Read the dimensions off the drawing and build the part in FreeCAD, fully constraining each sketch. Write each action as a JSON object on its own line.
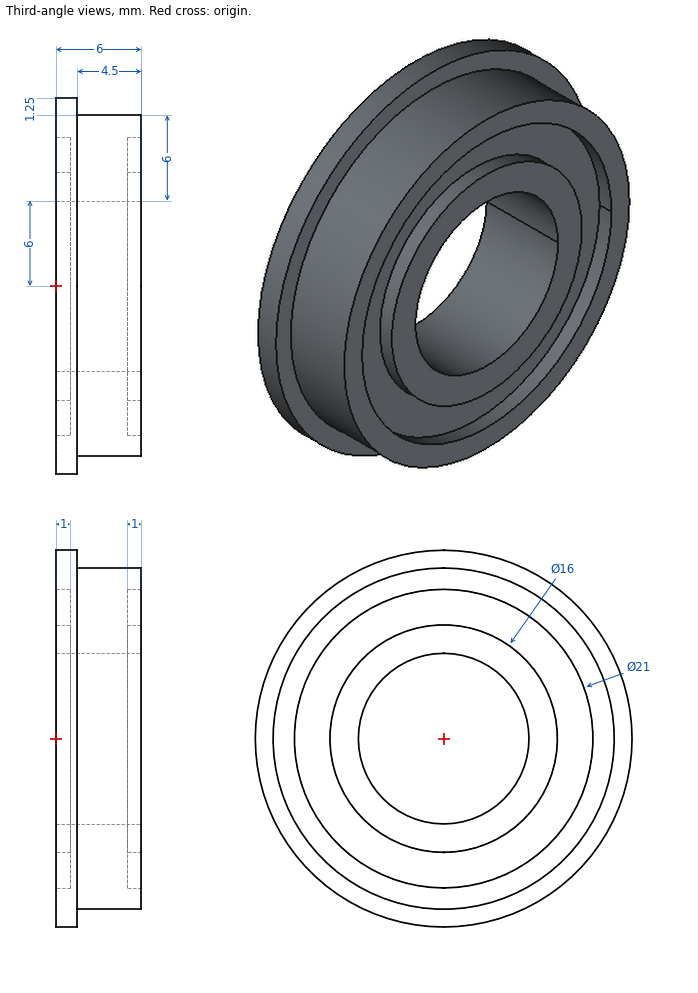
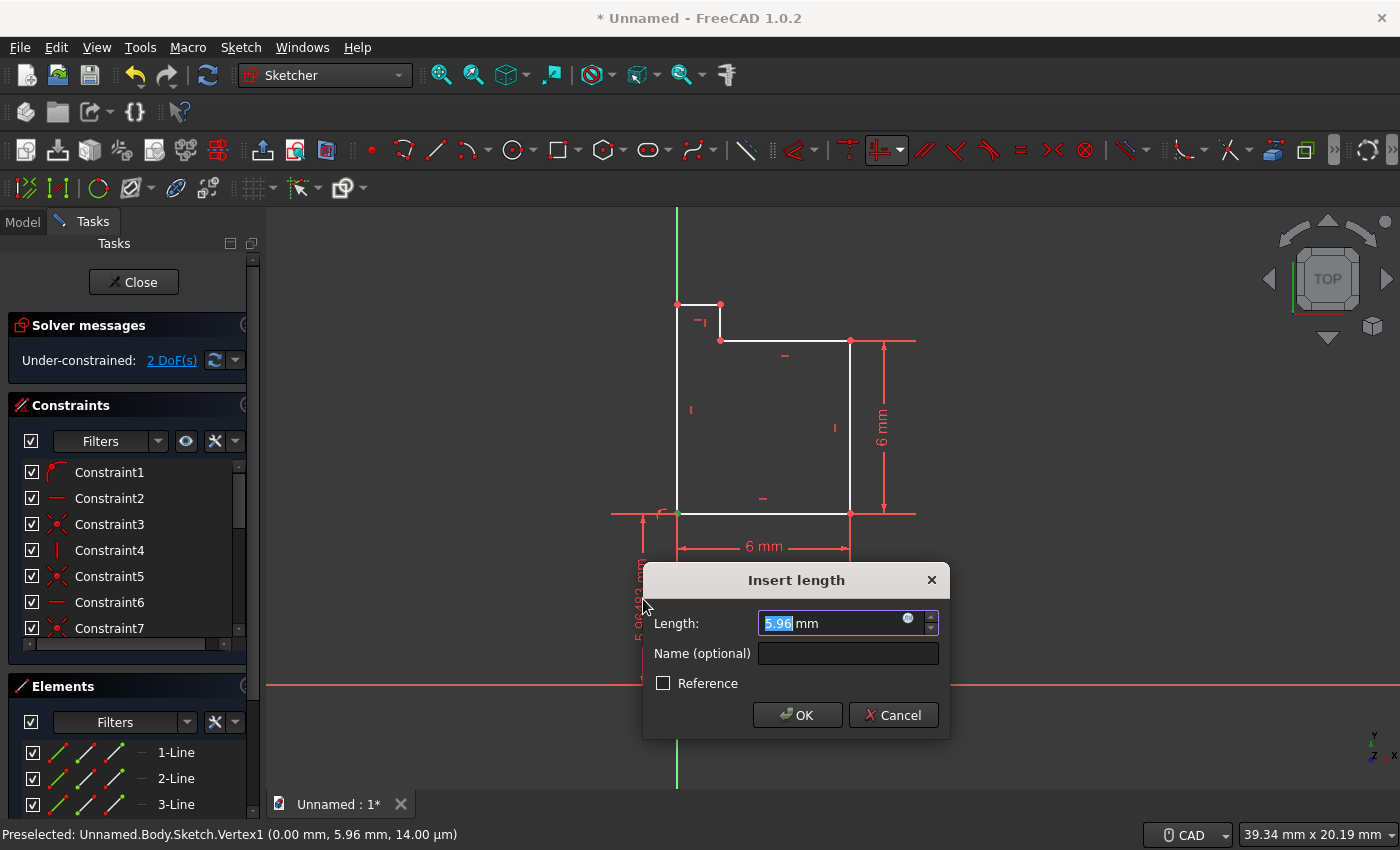
{"action": "type", "text": "6"}
{"action": "key", "text": "Return"}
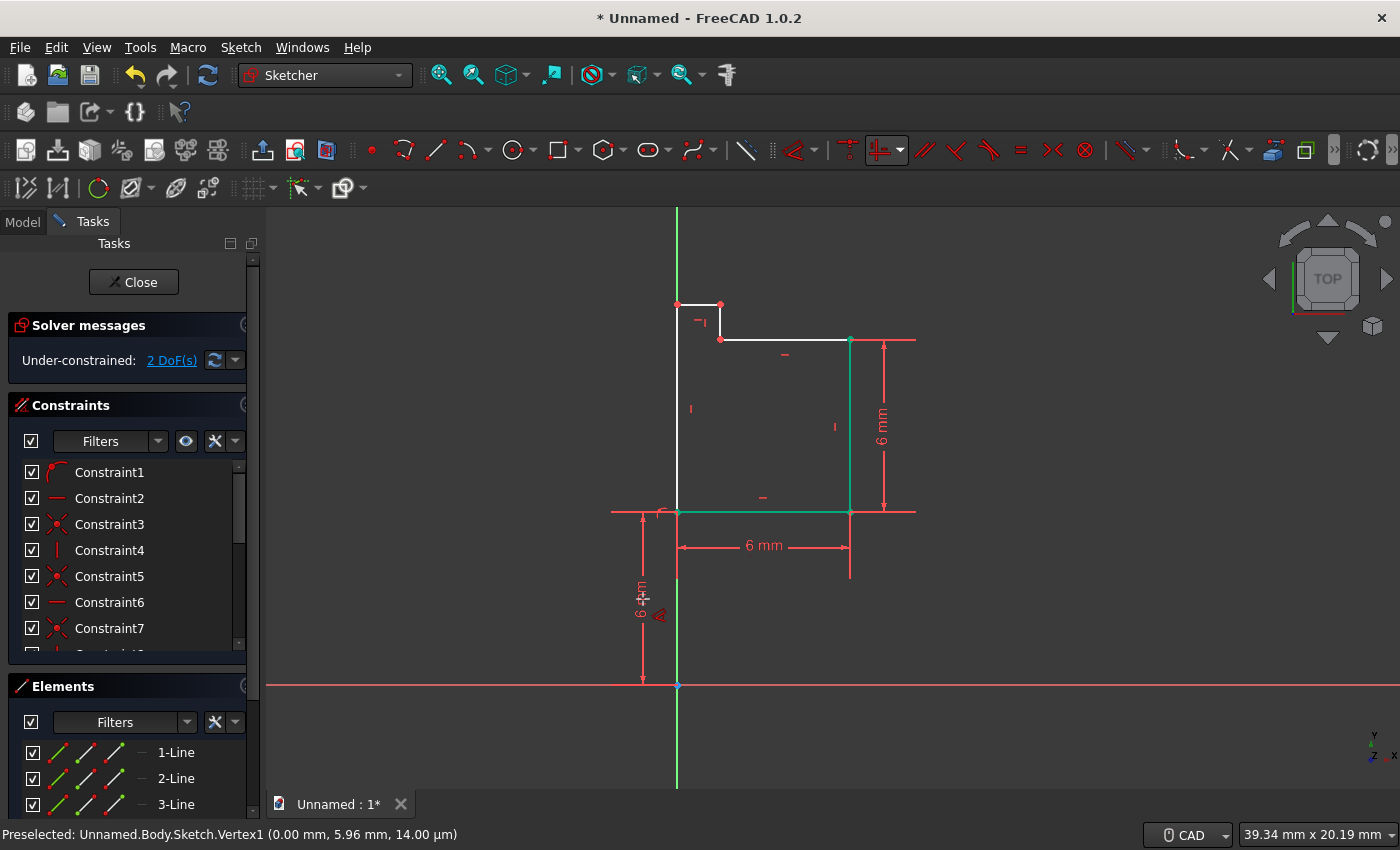
{"action": "left_click", "coordinate": [811, 340]}
{"action": "left_click", "coordinate": [785, 306]}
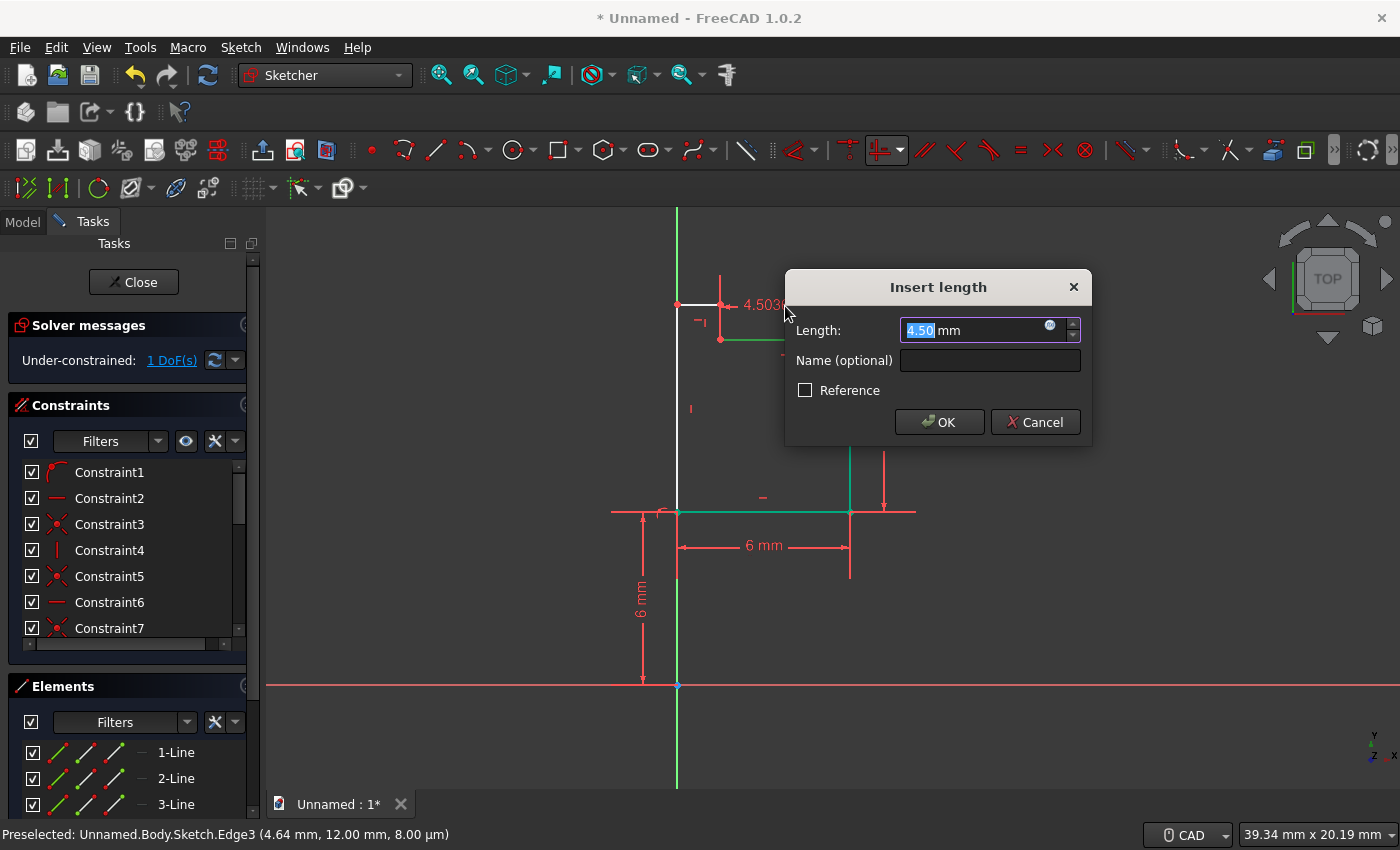
{"action": "type", "text": "4.5"}
{"action": "key", "text": "Return"}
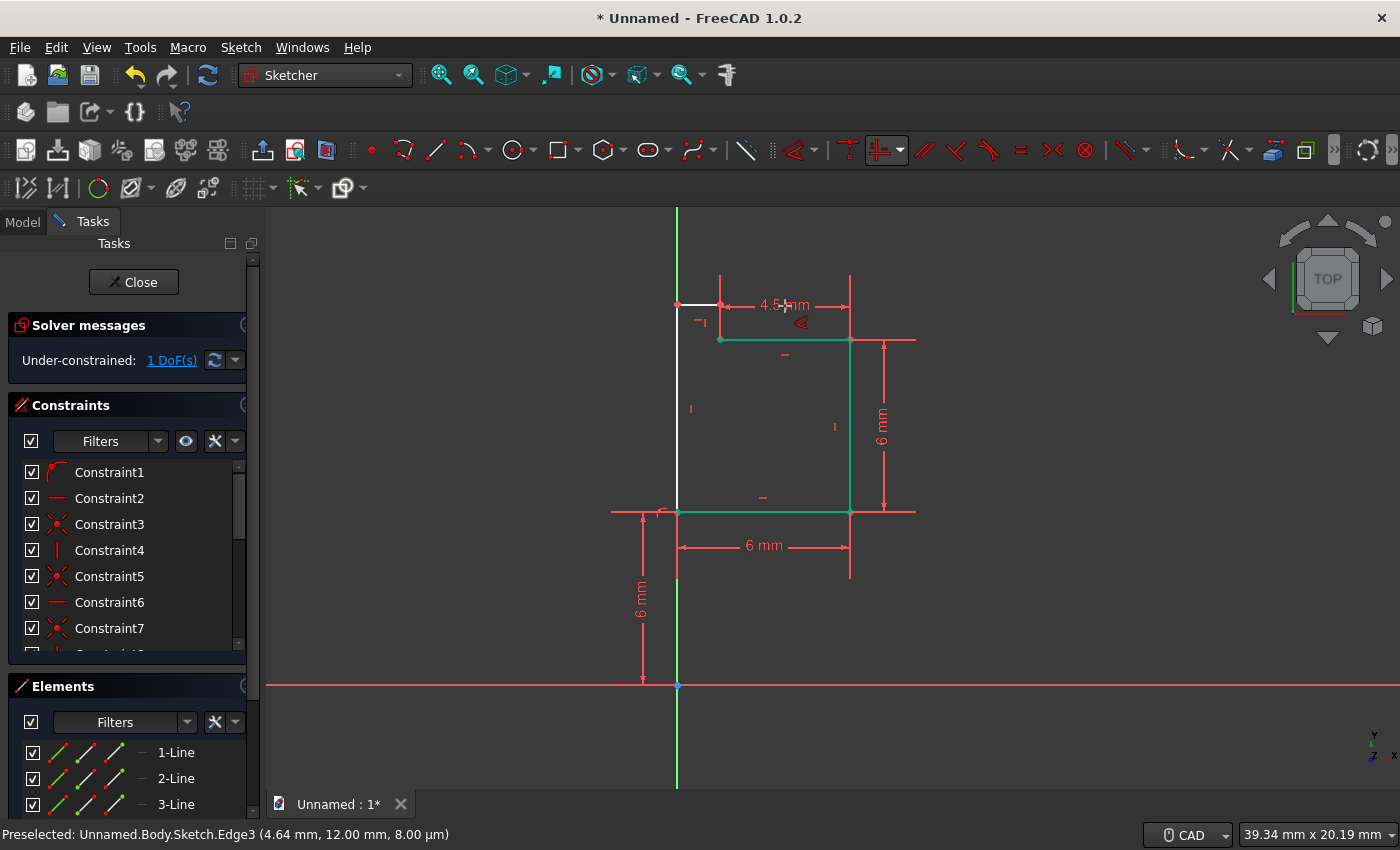
{"action": "scroll", "coordinate": [720, 329], "scroll_direction": "up", "scroll_amount": 2}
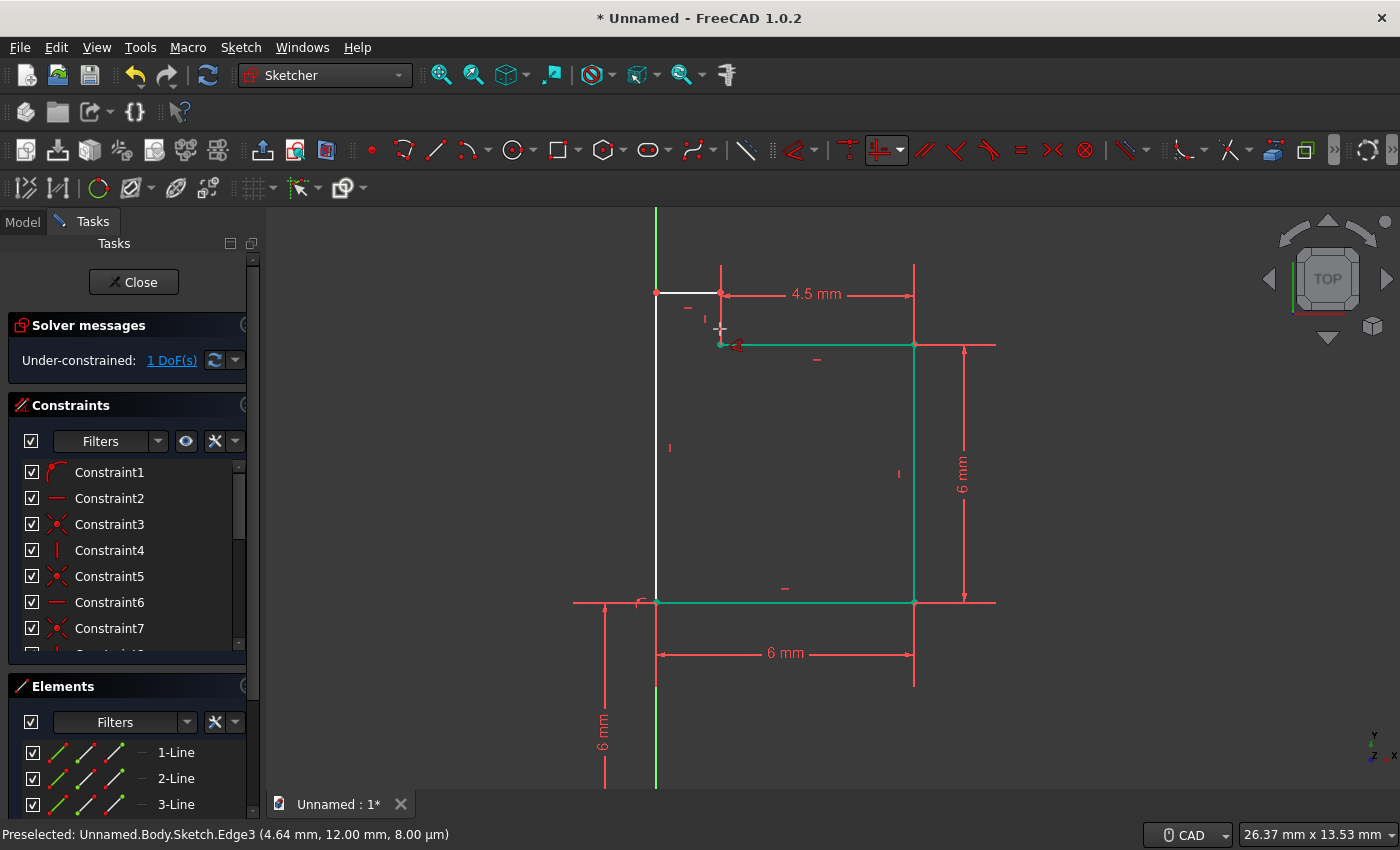
{"action": "left_click", "coordinate": [721, 329]}
{"action": "left_click", "coordinate": [687, 319]}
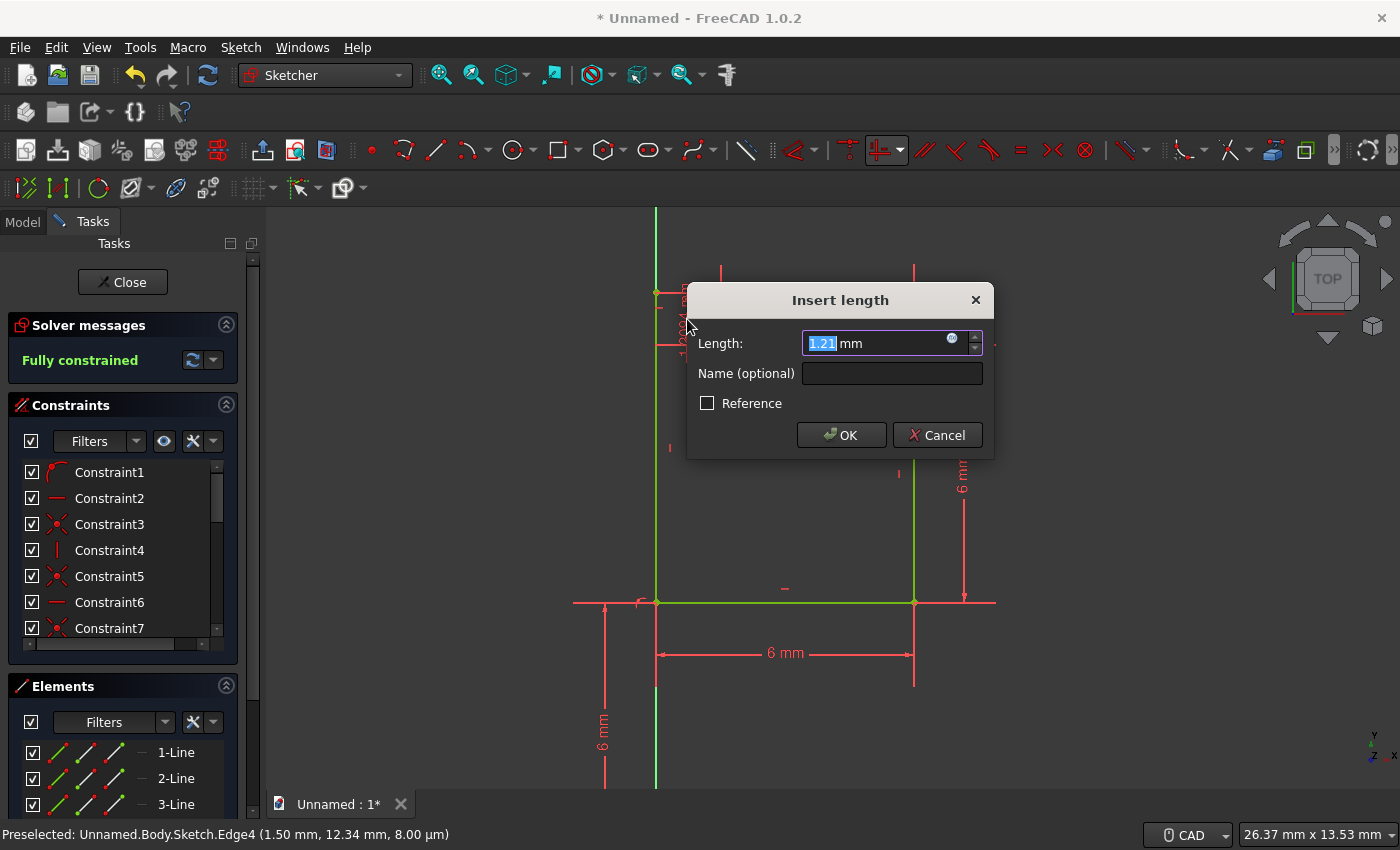
{"action": "type", "text": "1.25"}
{"action": "key", "text": "Return"}
{"action": "key", "text": "Escape"}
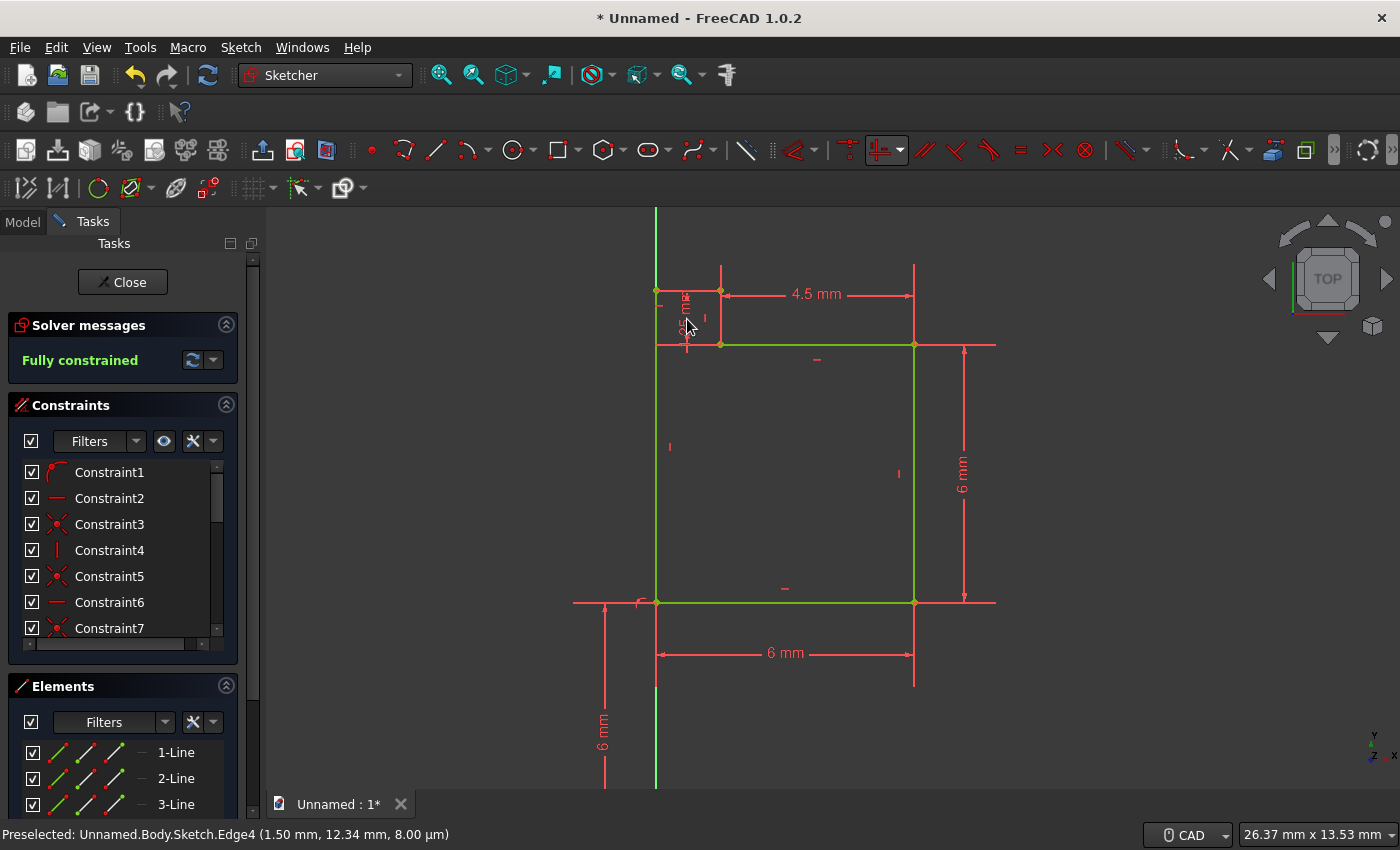
{"action": "left_click", "coordinate": [123, 282]}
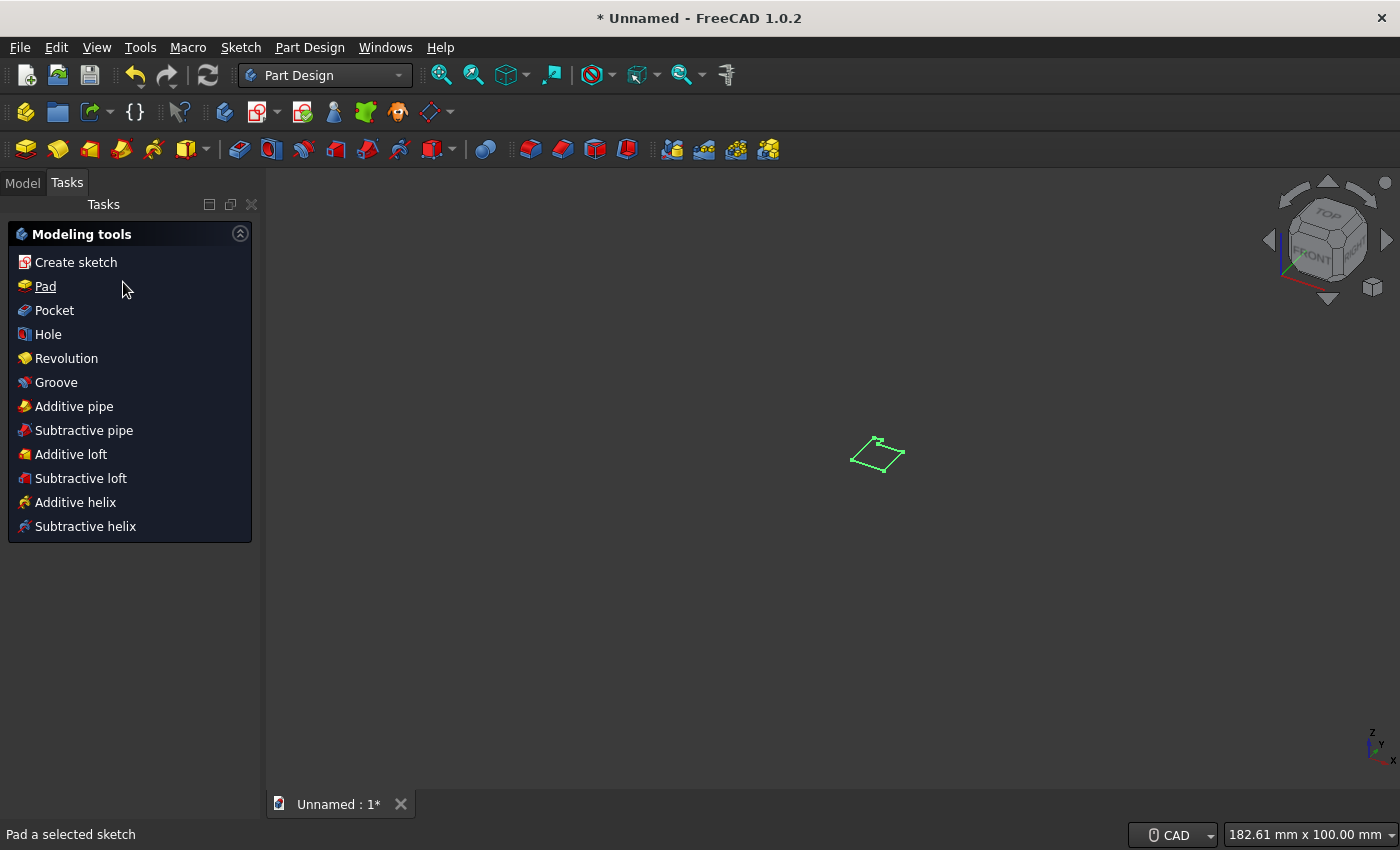
{"action": "left_click", "coordinate": [58, 150]}